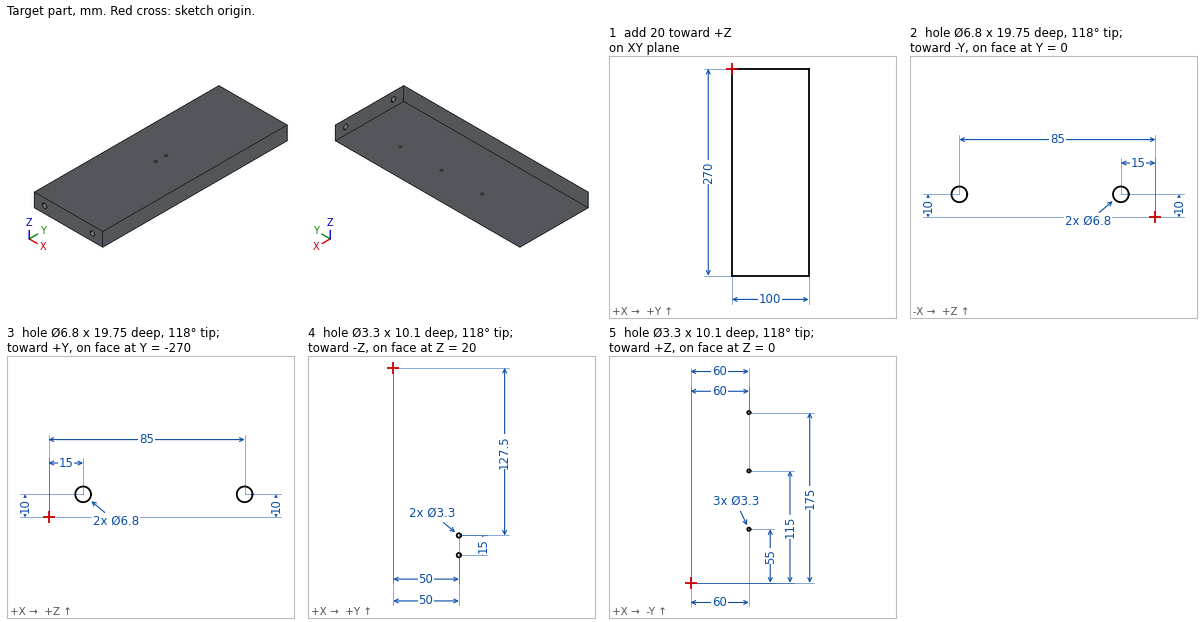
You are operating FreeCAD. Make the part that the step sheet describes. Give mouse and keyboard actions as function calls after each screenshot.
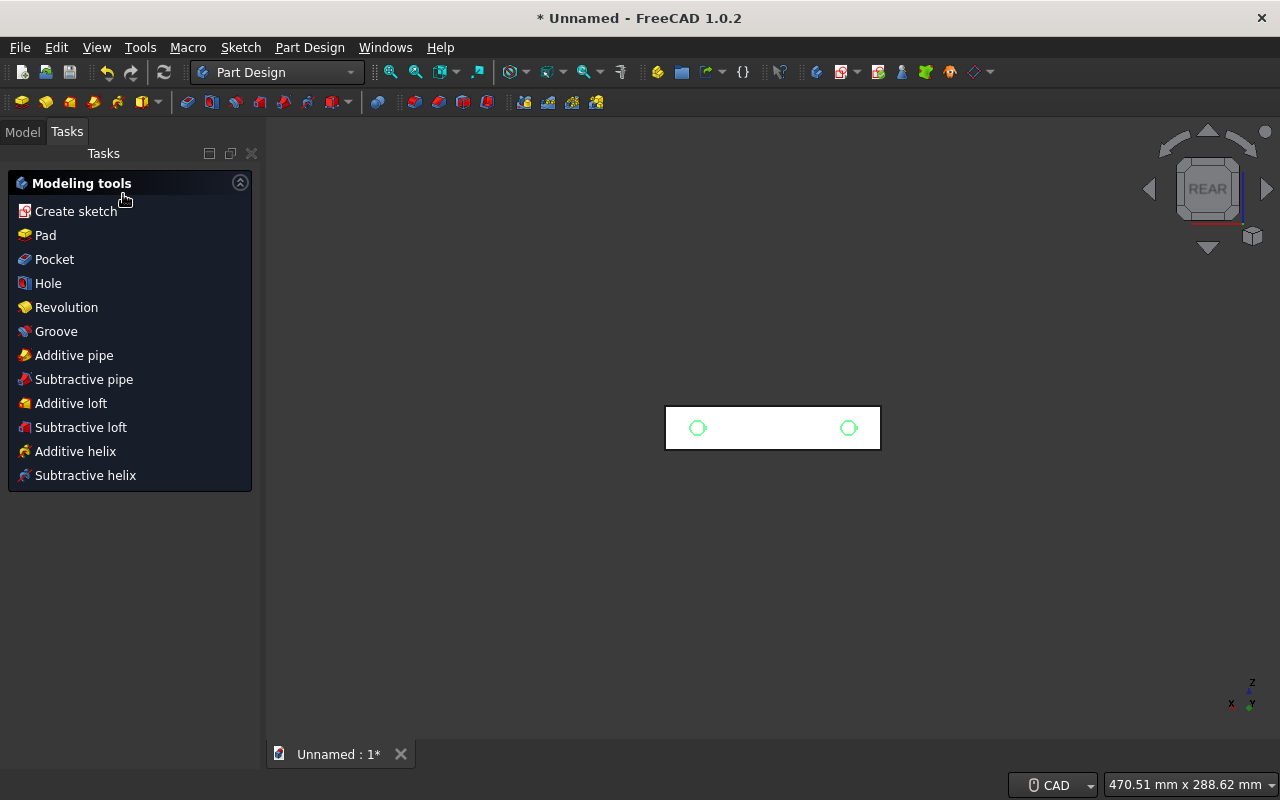
click(212, 102)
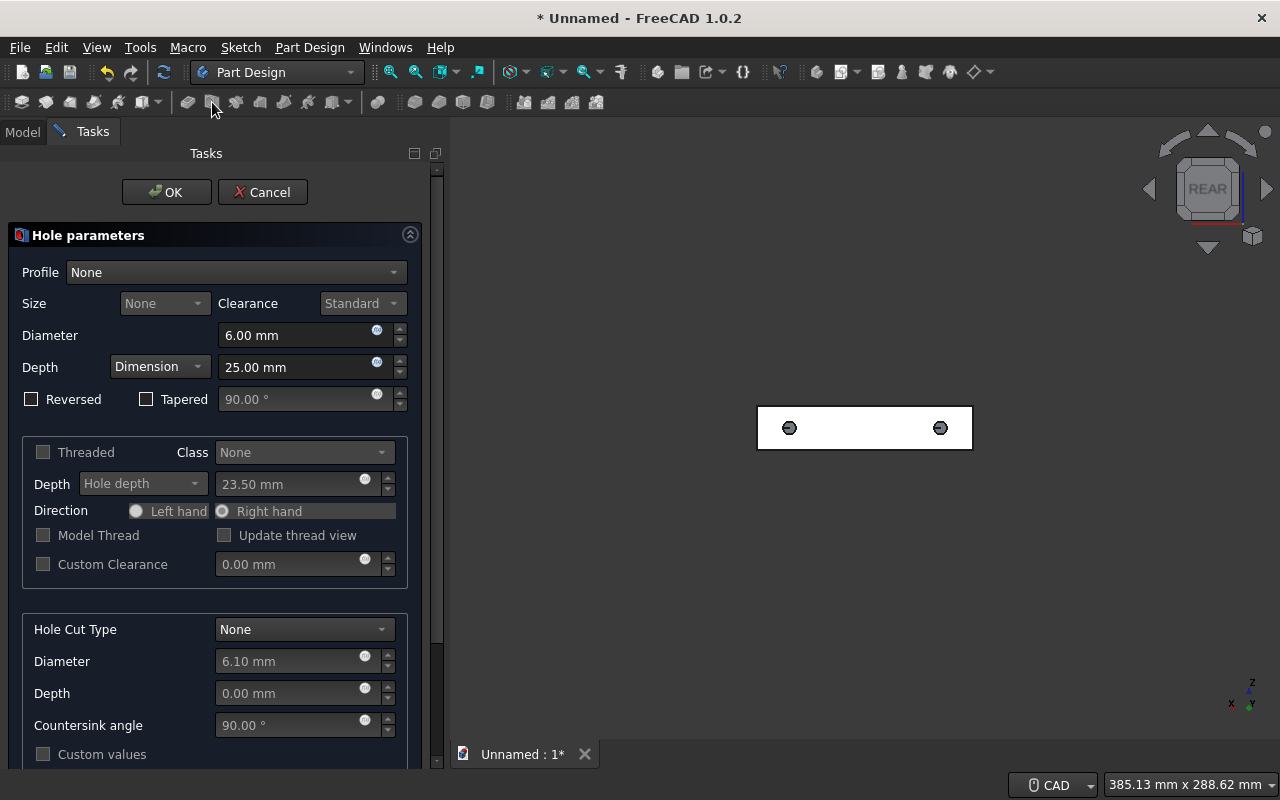
triple_click(305, 335)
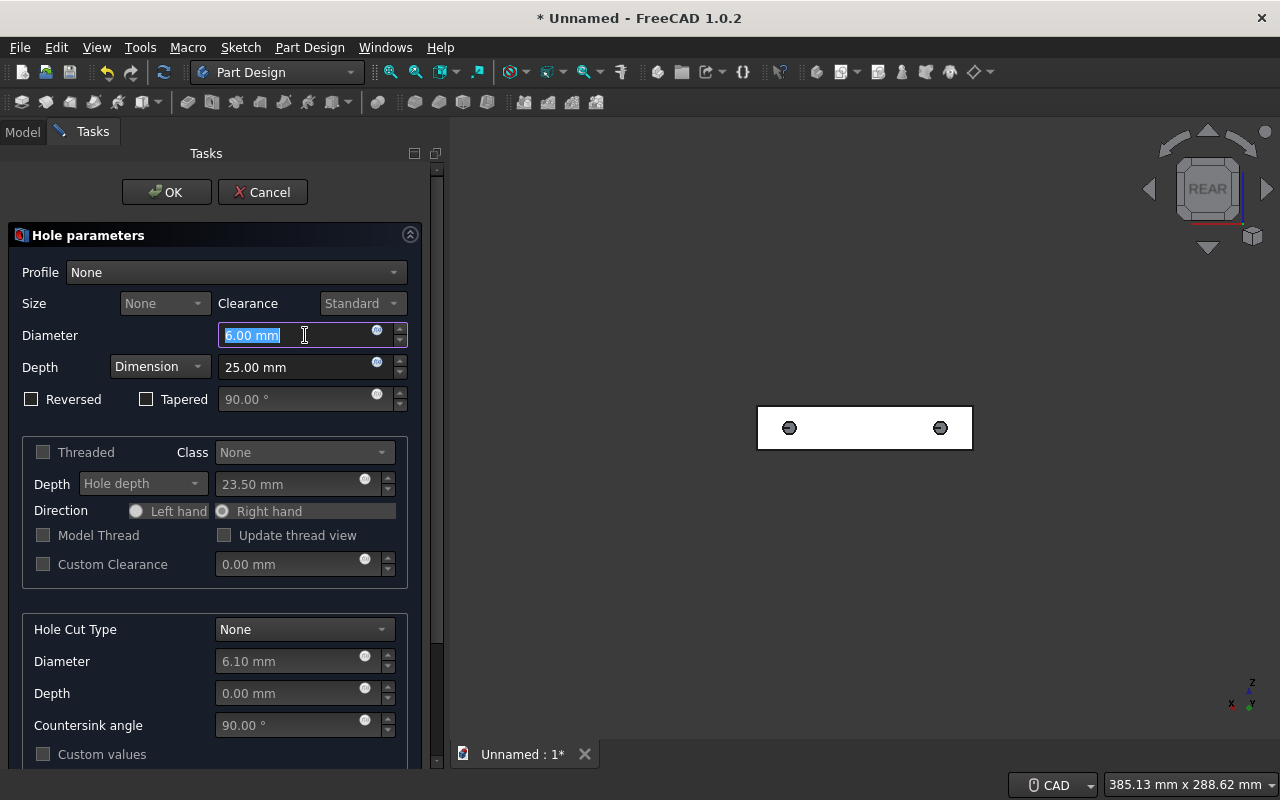
text(6.8)
key(Tab)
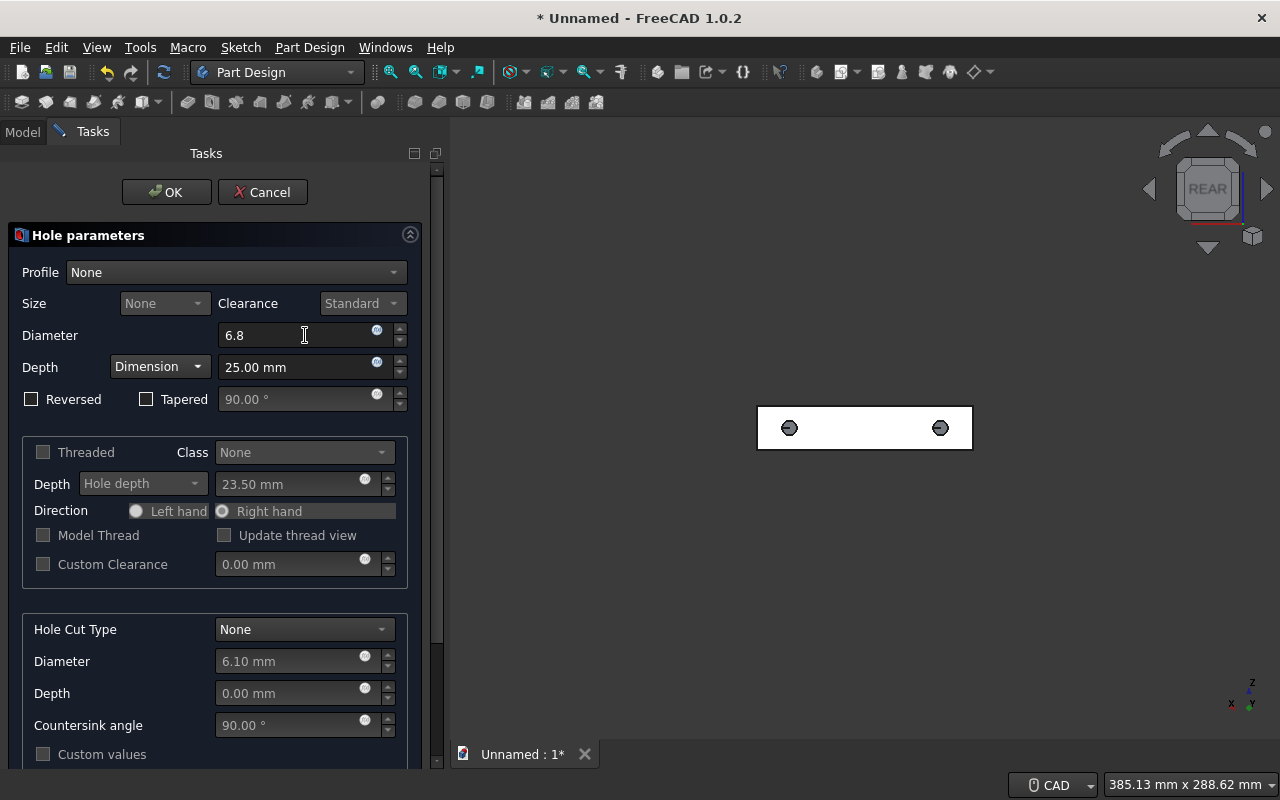
triple_click(305, 367)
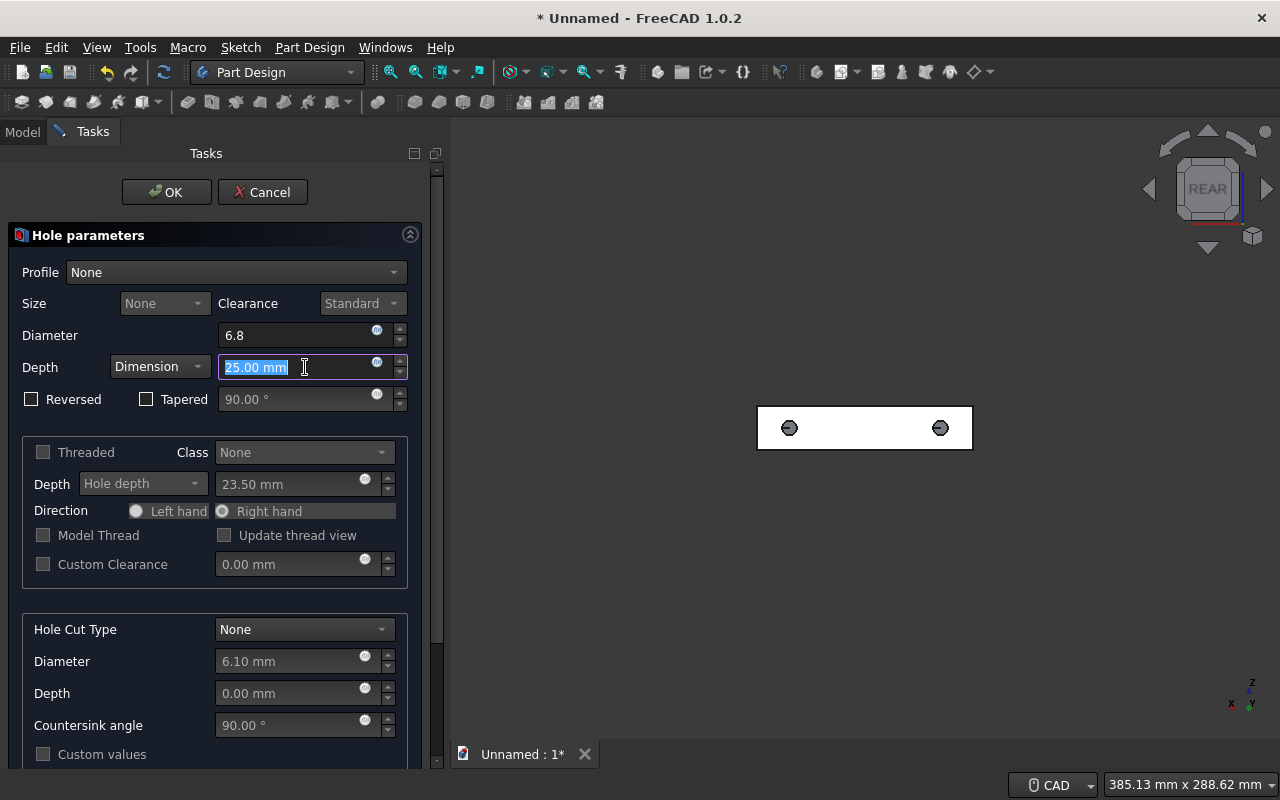
text(19.75)
key(Tab)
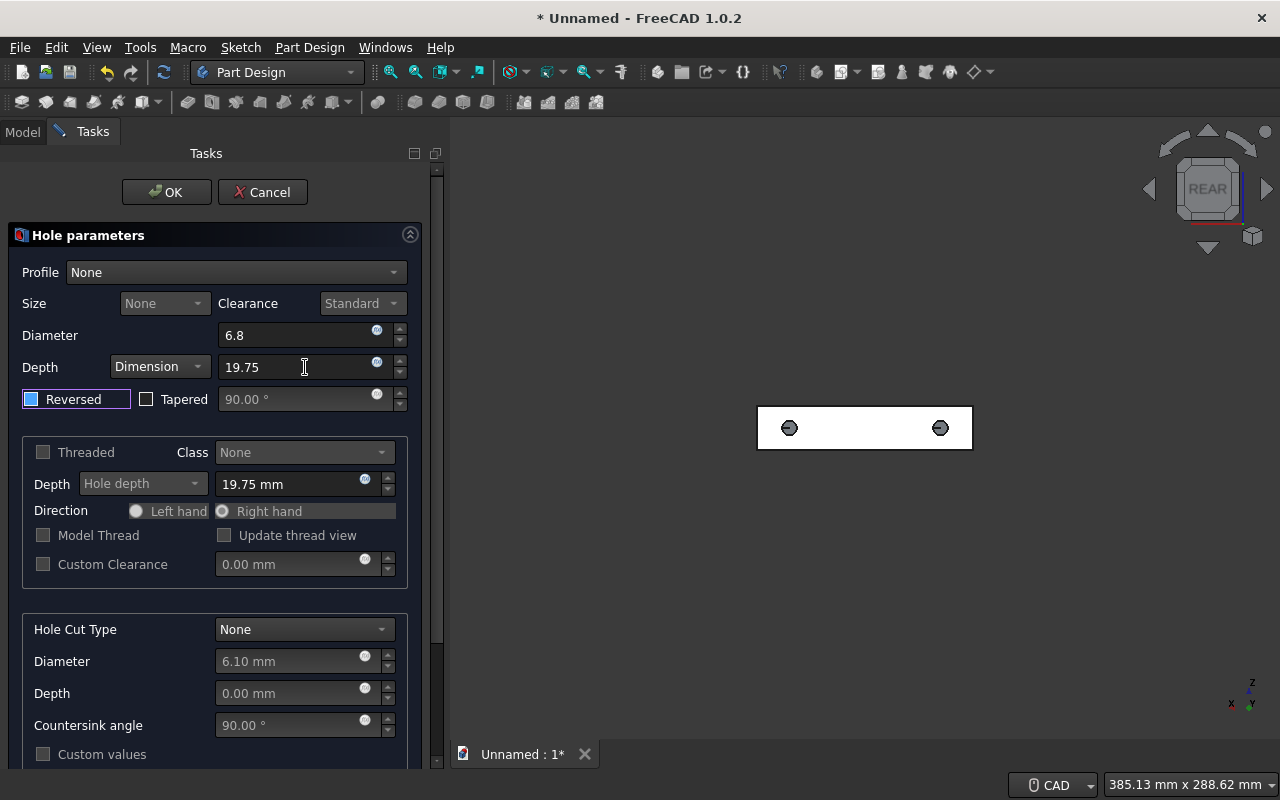
click(167, 192)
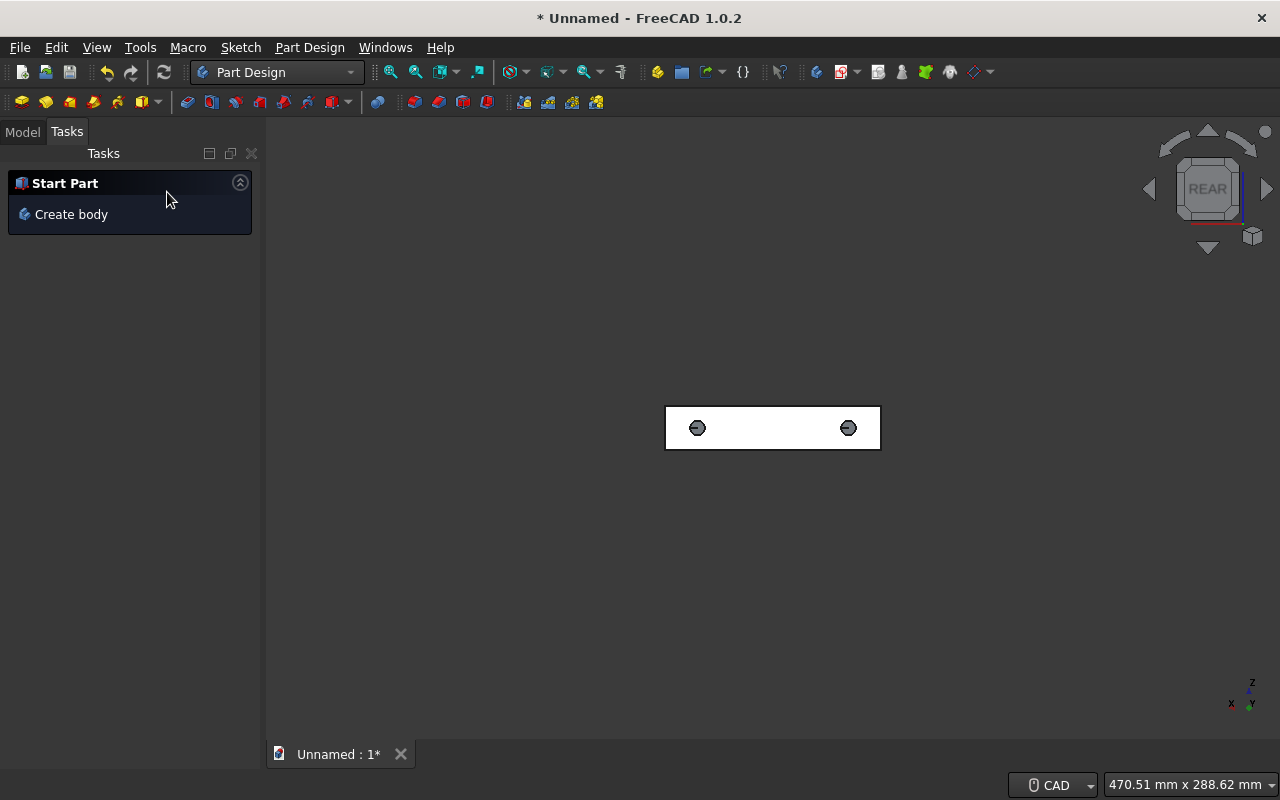
click(392, 72)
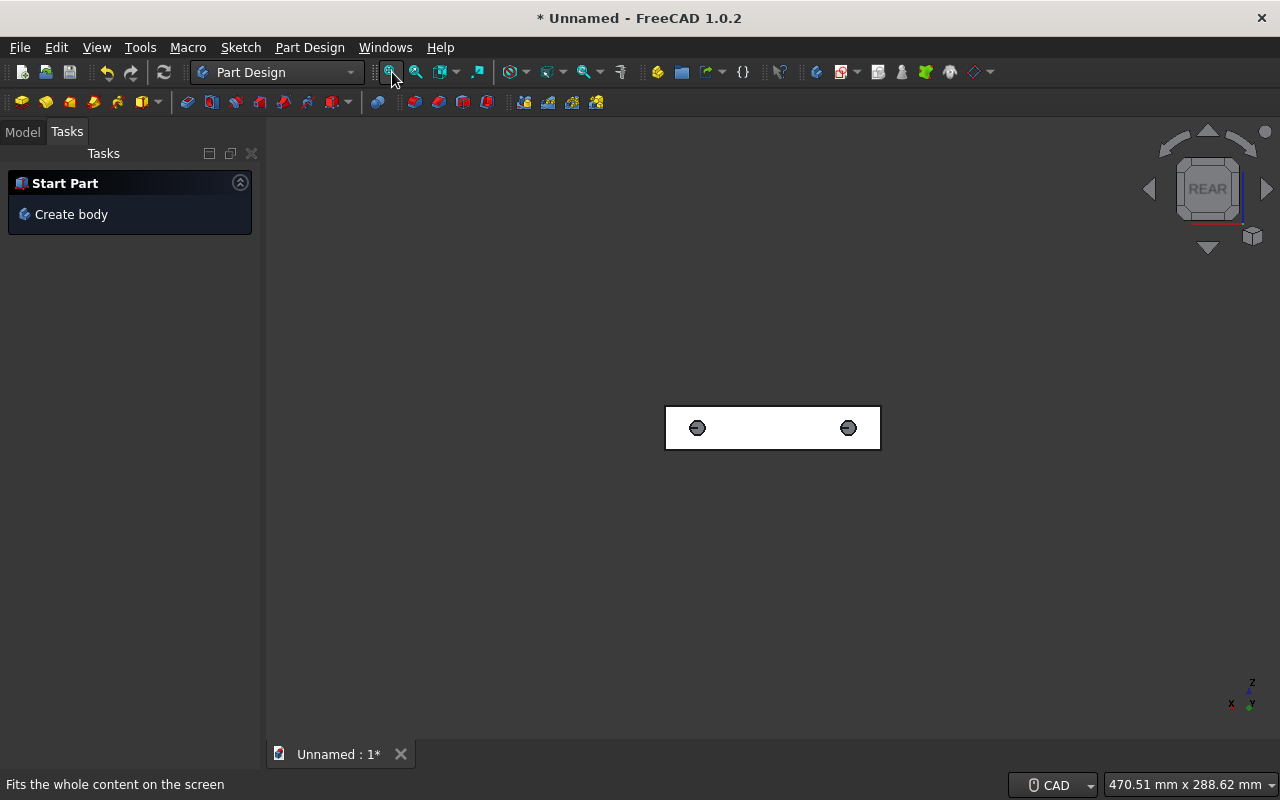
key(0)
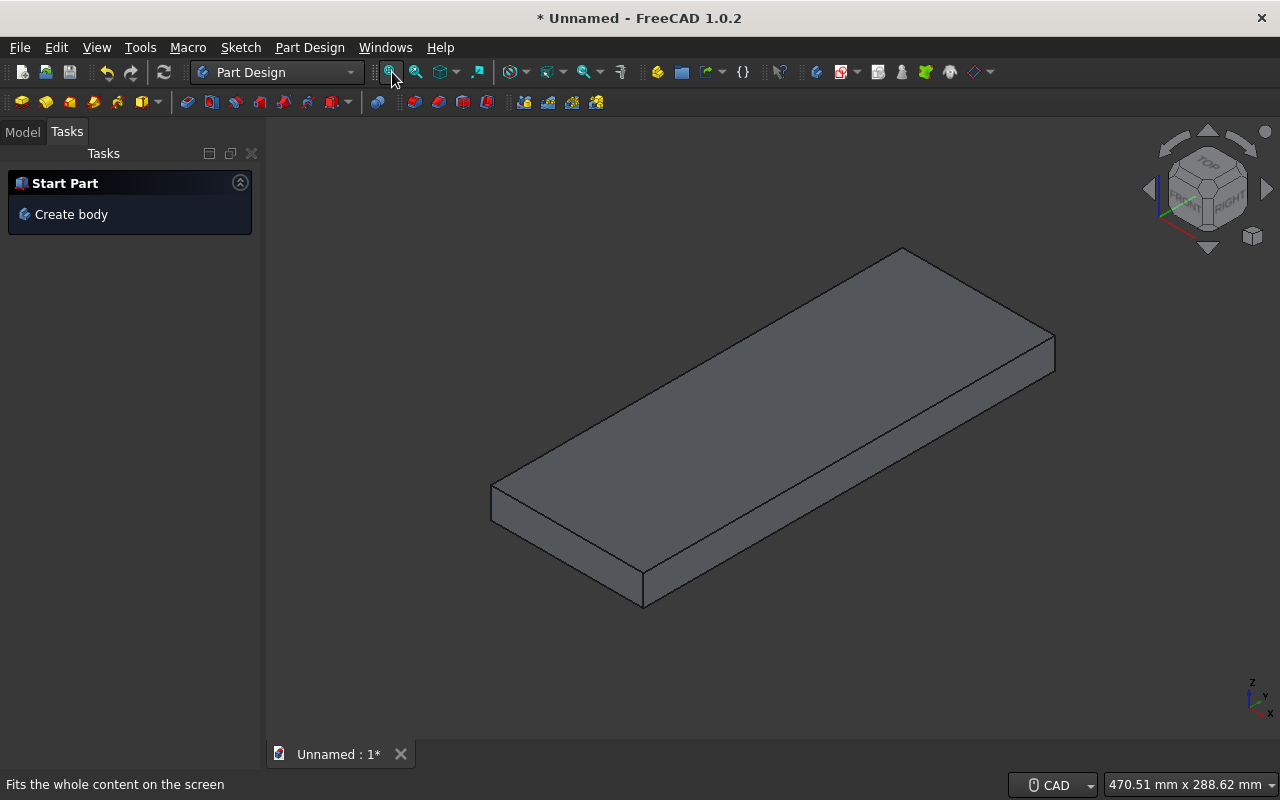
click(611, 571)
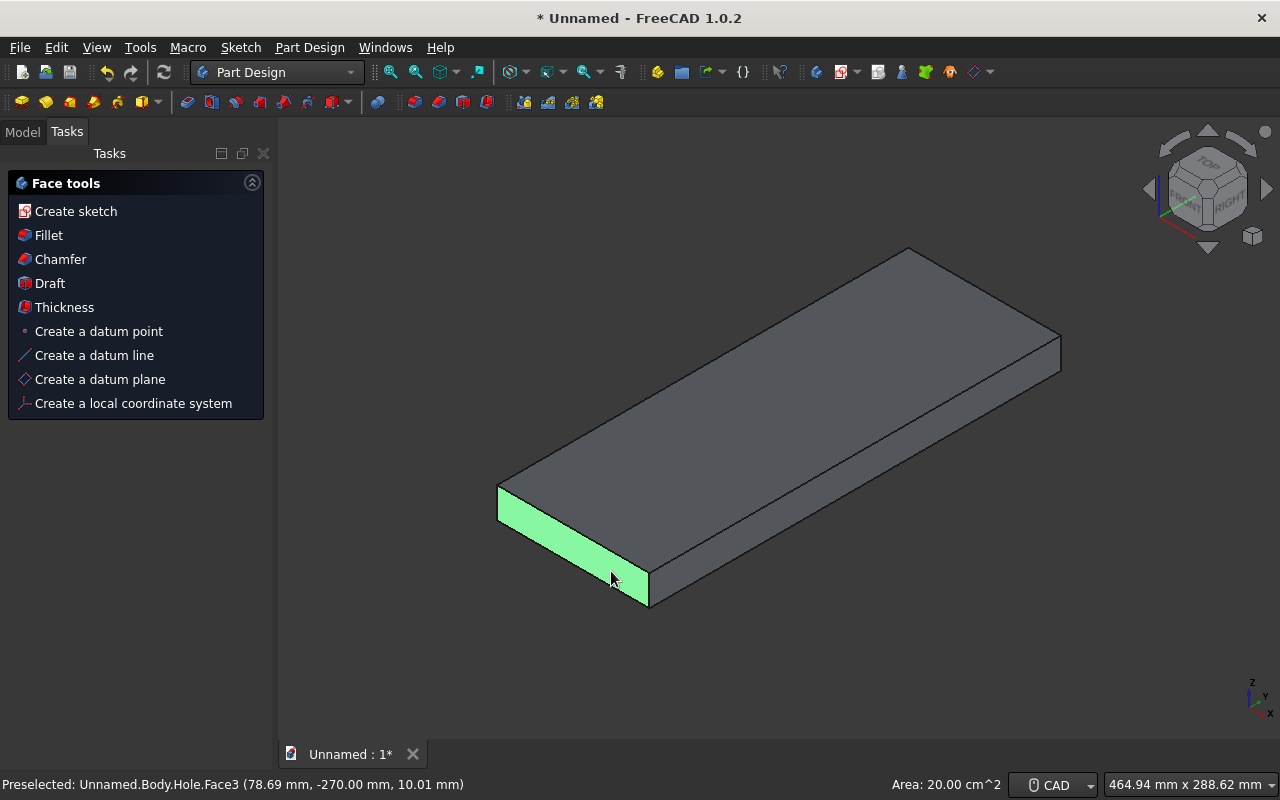
click(842, 72)